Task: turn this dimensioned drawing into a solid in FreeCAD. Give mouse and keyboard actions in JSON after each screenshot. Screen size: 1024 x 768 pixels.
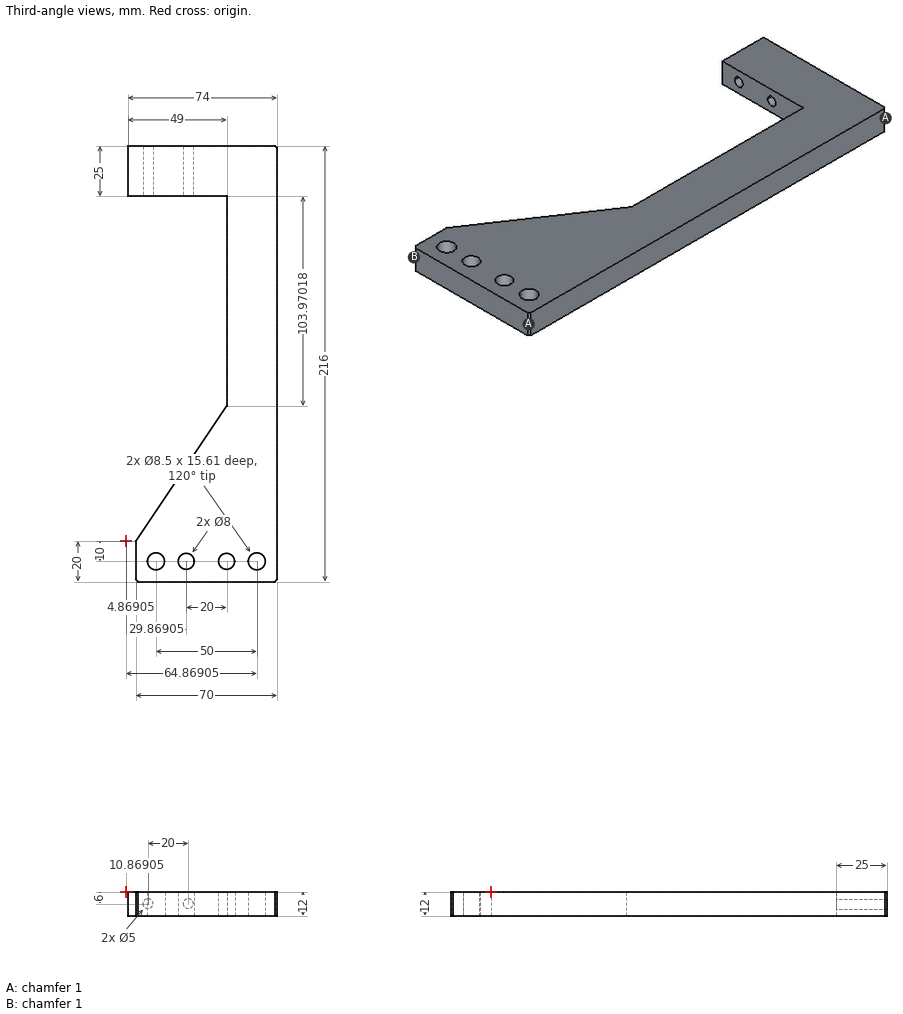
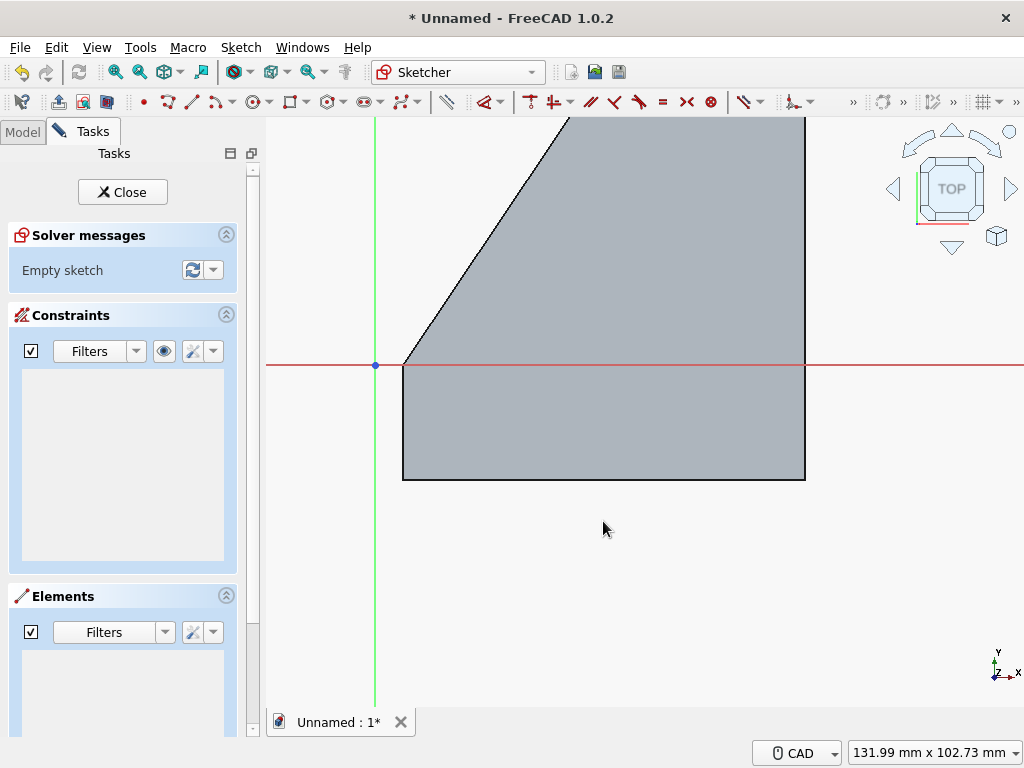
{"action": "key", "text": "g c"}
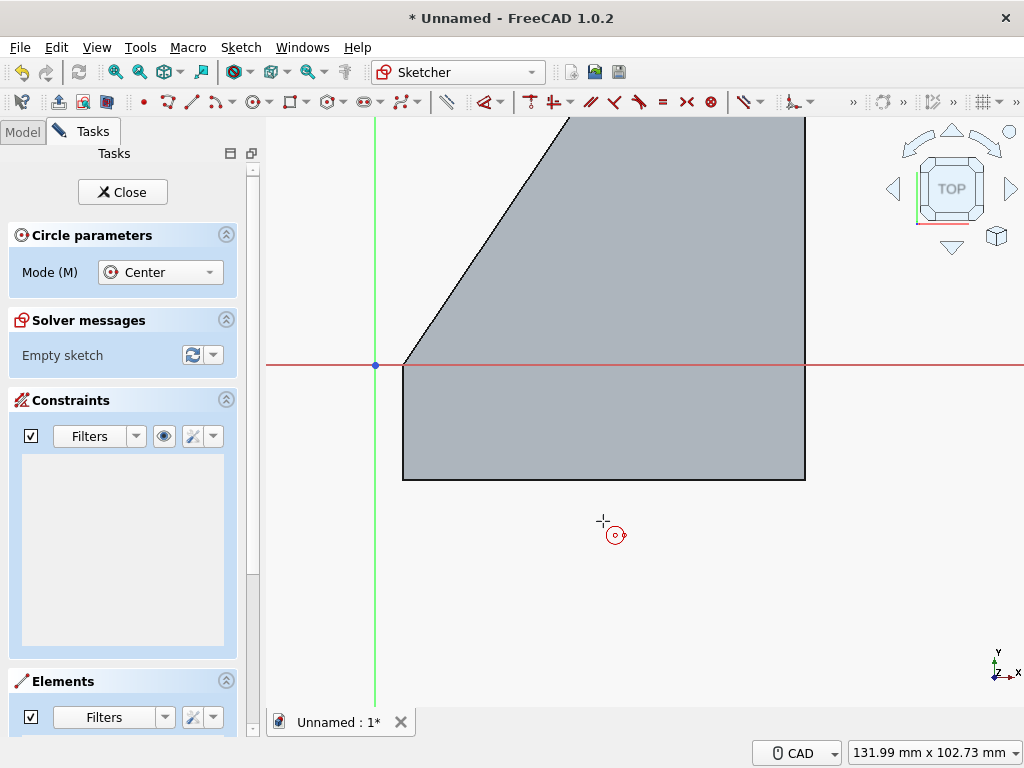
{"action": "left_click", "coordinate": [748, 423]}
{"action": "left_click", "coordinate": [765, 406]}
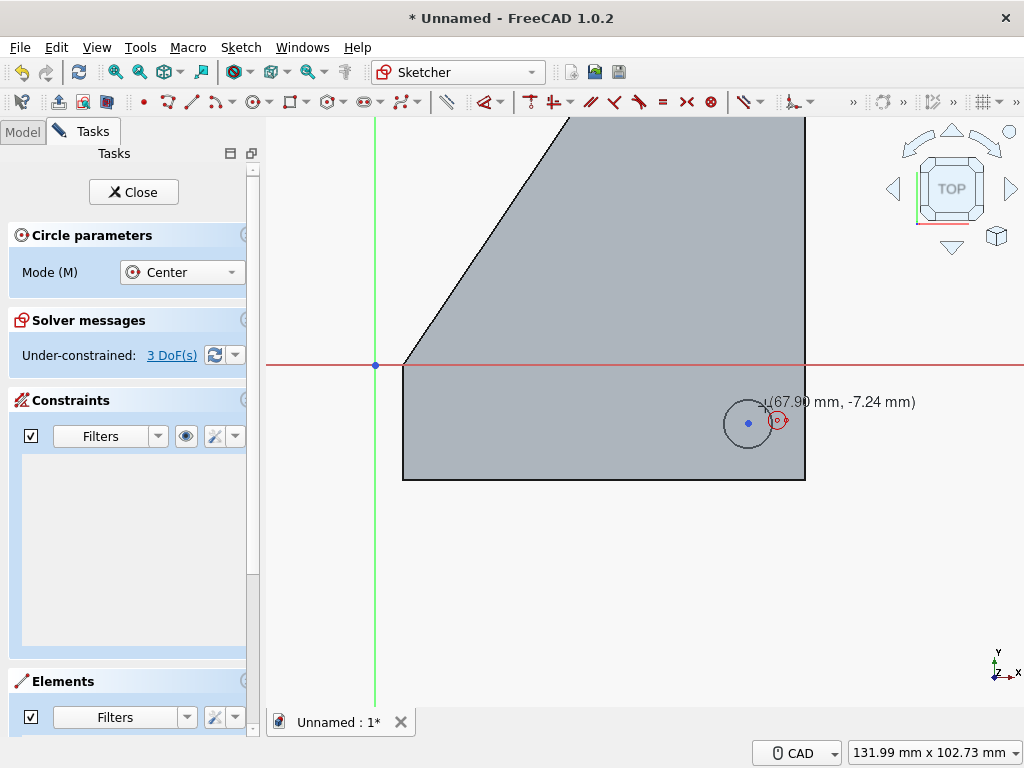
{"action": "left_click", "coordinate": [460, 423]}
{"action": "left_click", "coordinate": [478, 406]}
{"action": "key", "text": "Escape"}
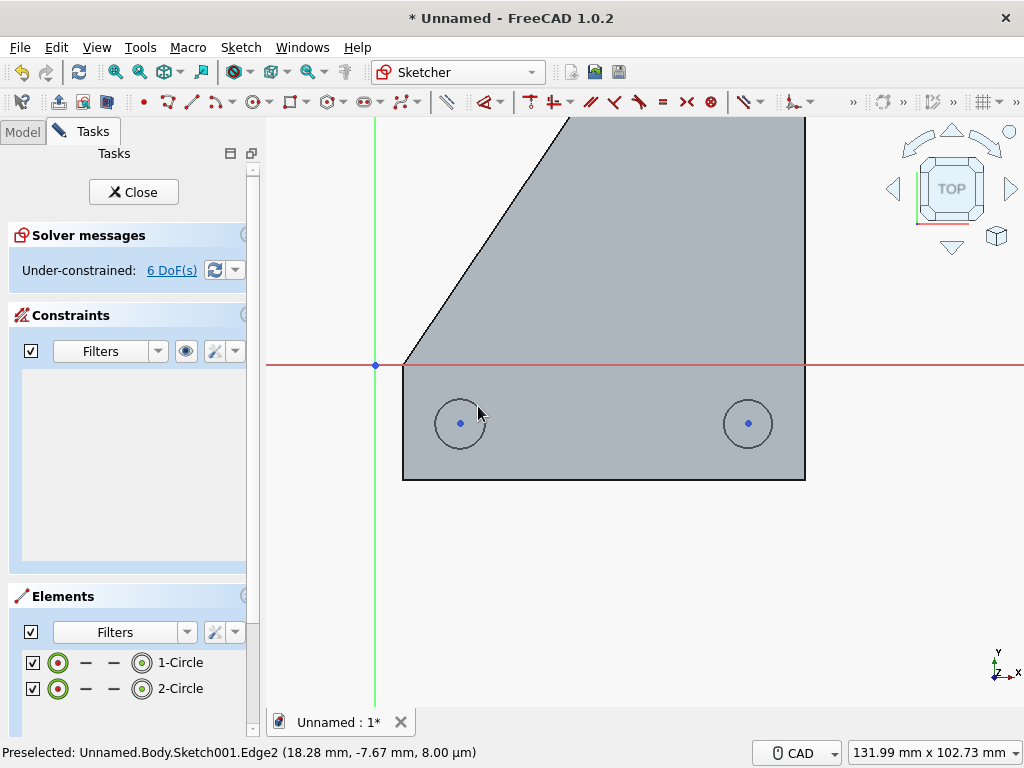
{"action": "left_click", "coordinate": [765, 407]}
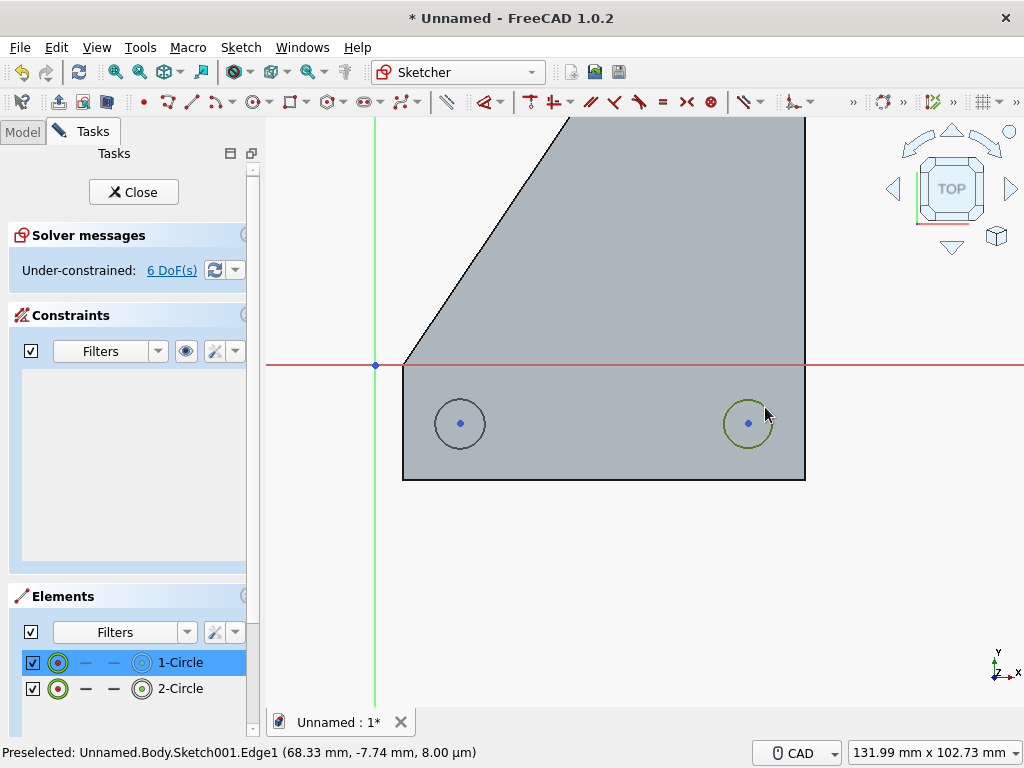
{"action": "left_click", "coordinate": [477, 406]}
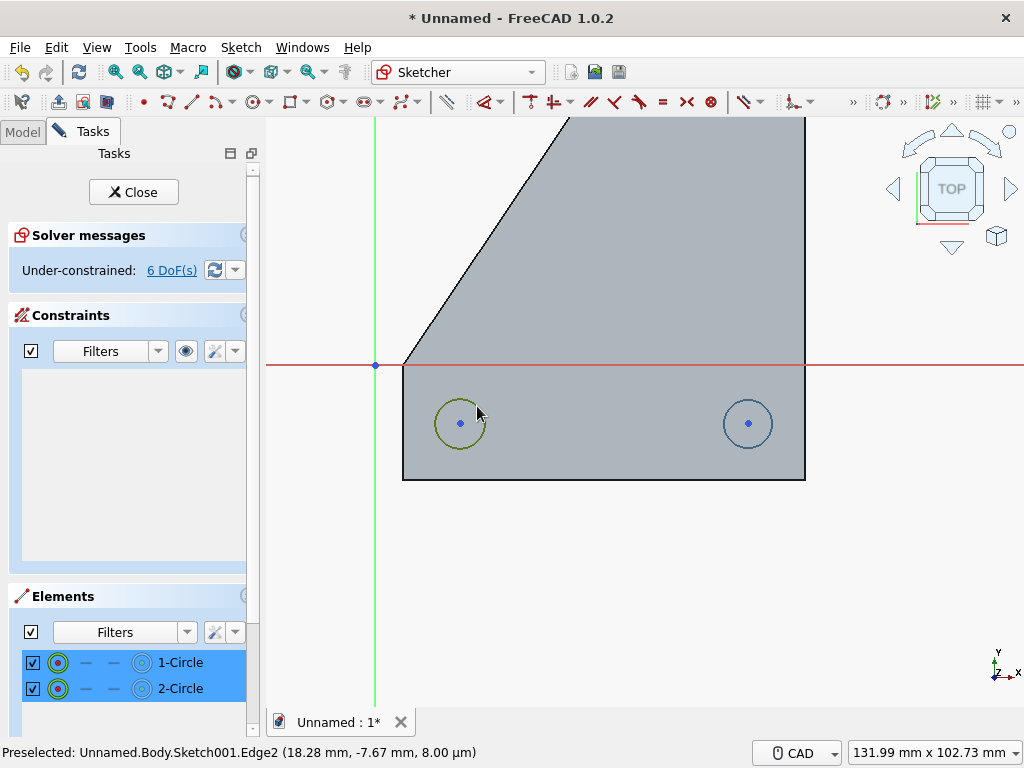
{"action": "key", "text": "e"}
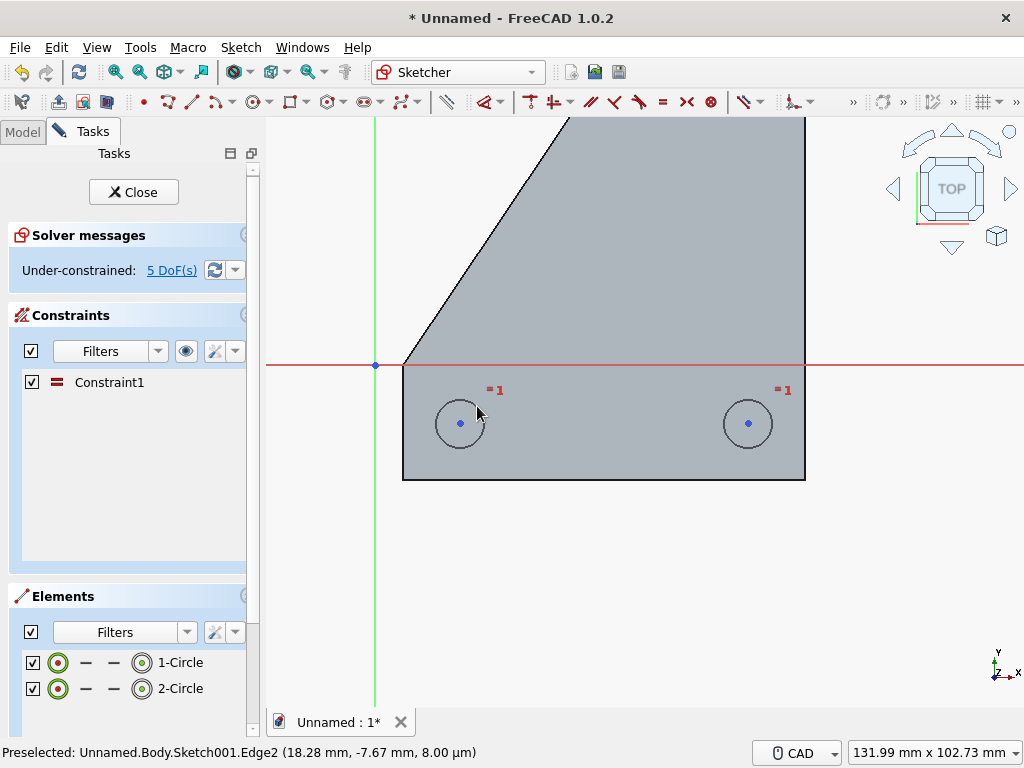
{"action": "key", "text": "d"}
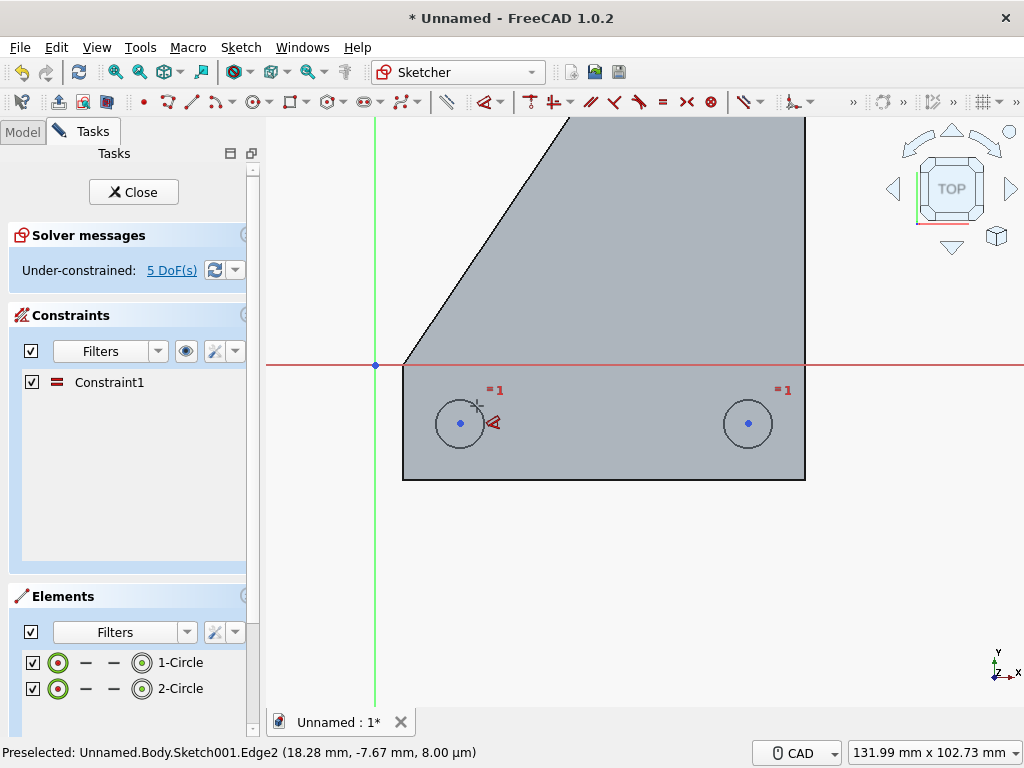
{"action": "left_click", "coordinate": [765, 407]}
{"action": "left_click", "coordinate": [788, 384]}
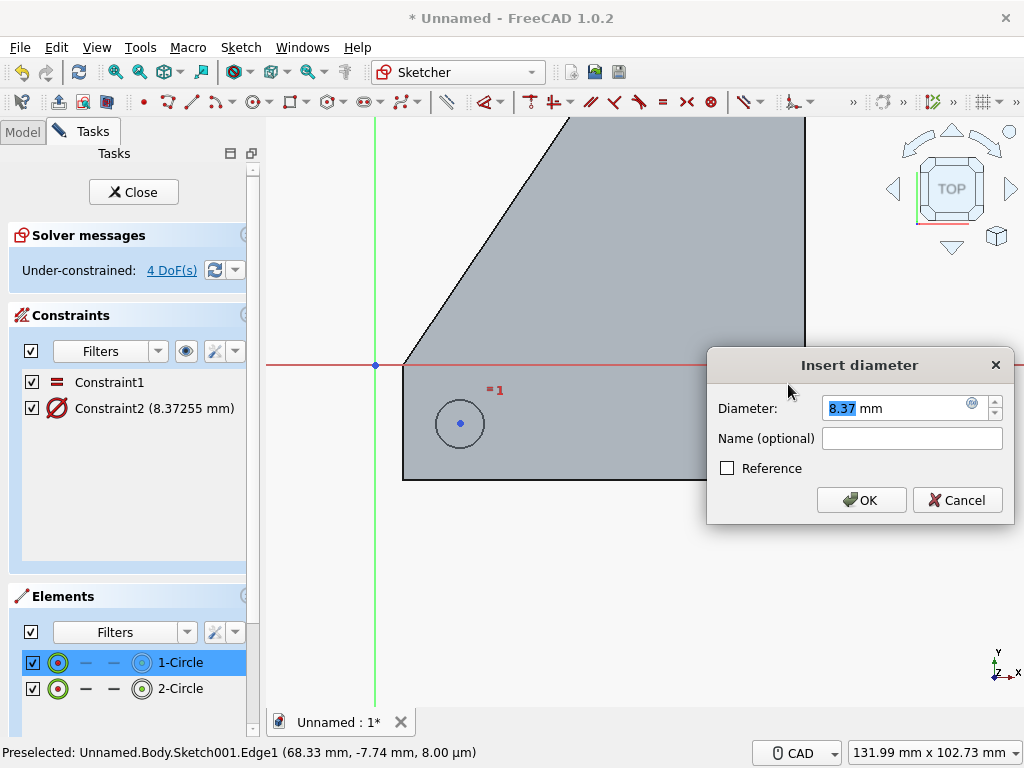
{"action": "type", "text": "8.5"}
{"action": "key", "text": "Return"}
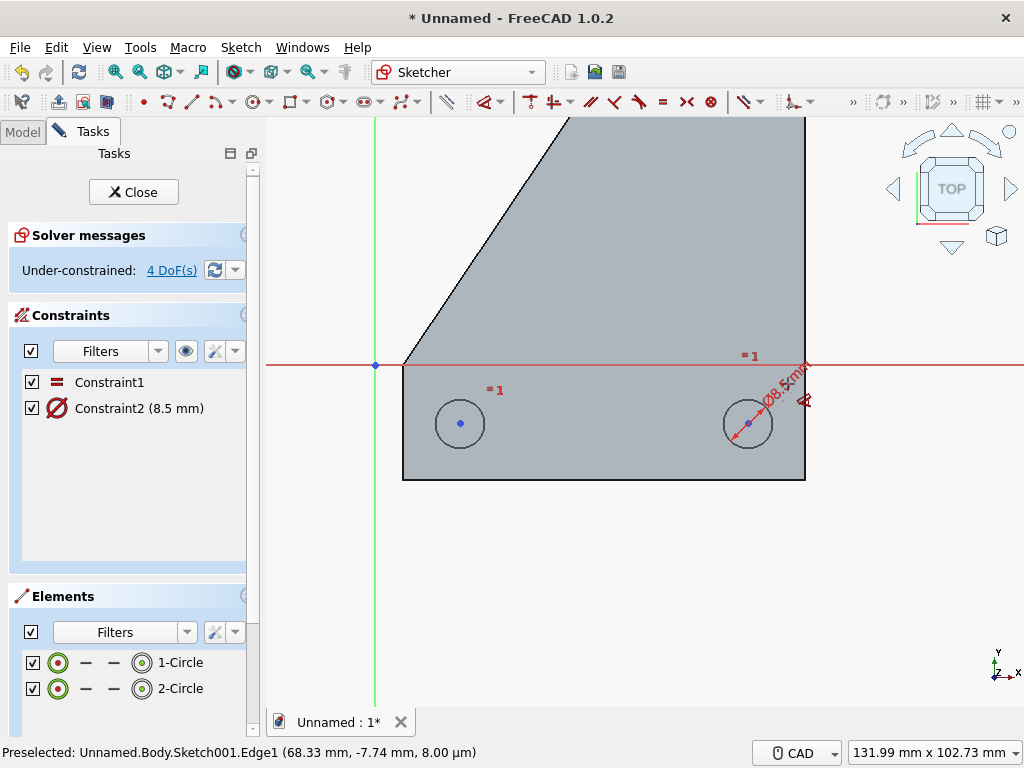
{"action": "left_click", "coordinate": [748, 424]}
{"action": "left_click", "coordinate": [341, 395]}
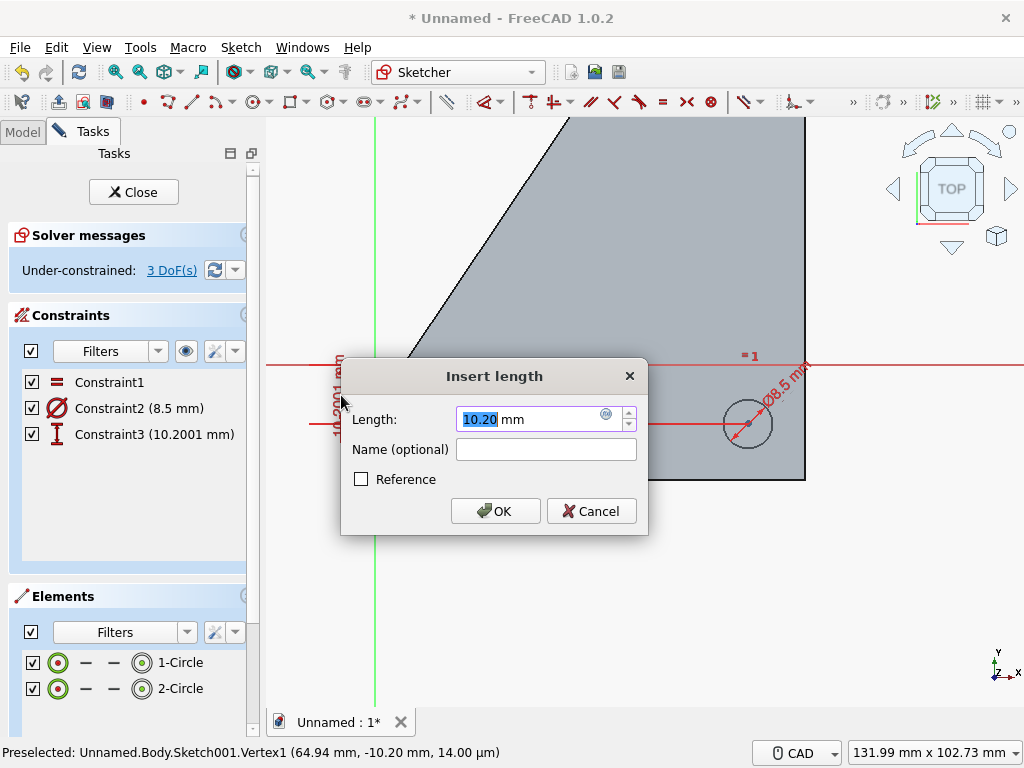
{"action": "type", "text": "10"}
{"action": "key", "text": "Return"}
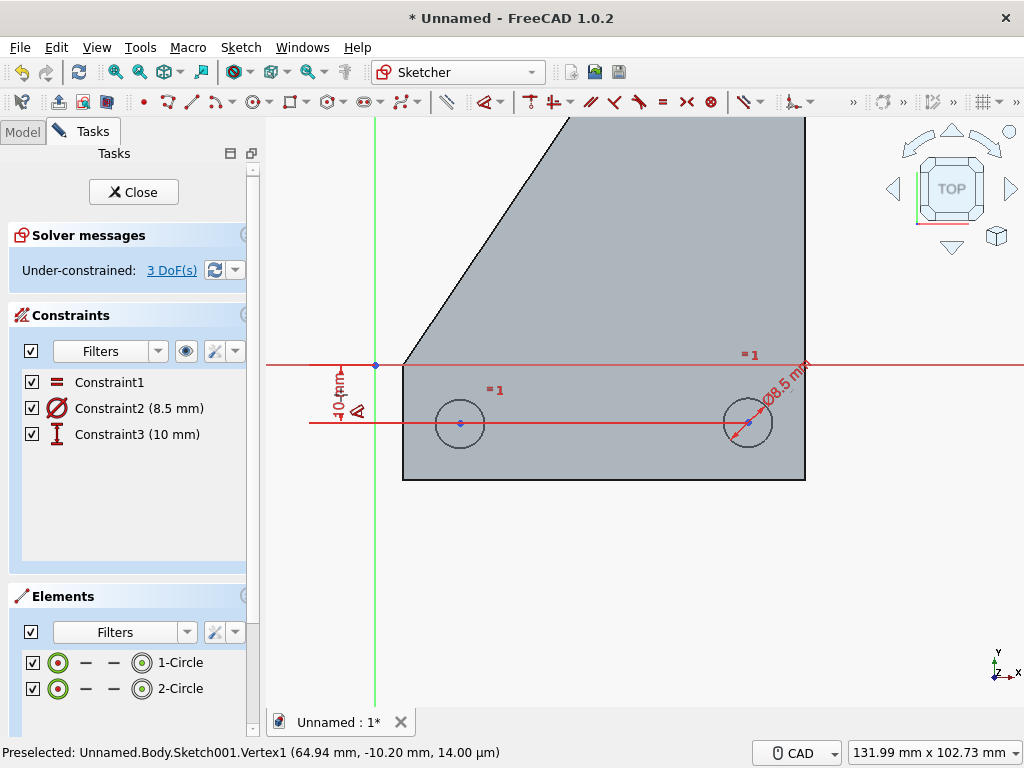
{"action": "left_click", "coordinate": [460, 424]}
{"action": "left_click", "coordinate": [341, 415]}